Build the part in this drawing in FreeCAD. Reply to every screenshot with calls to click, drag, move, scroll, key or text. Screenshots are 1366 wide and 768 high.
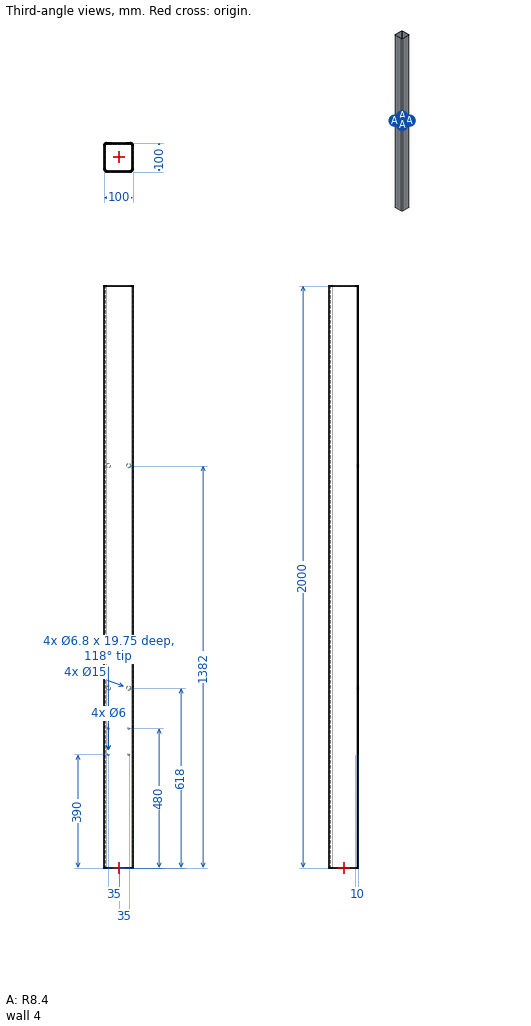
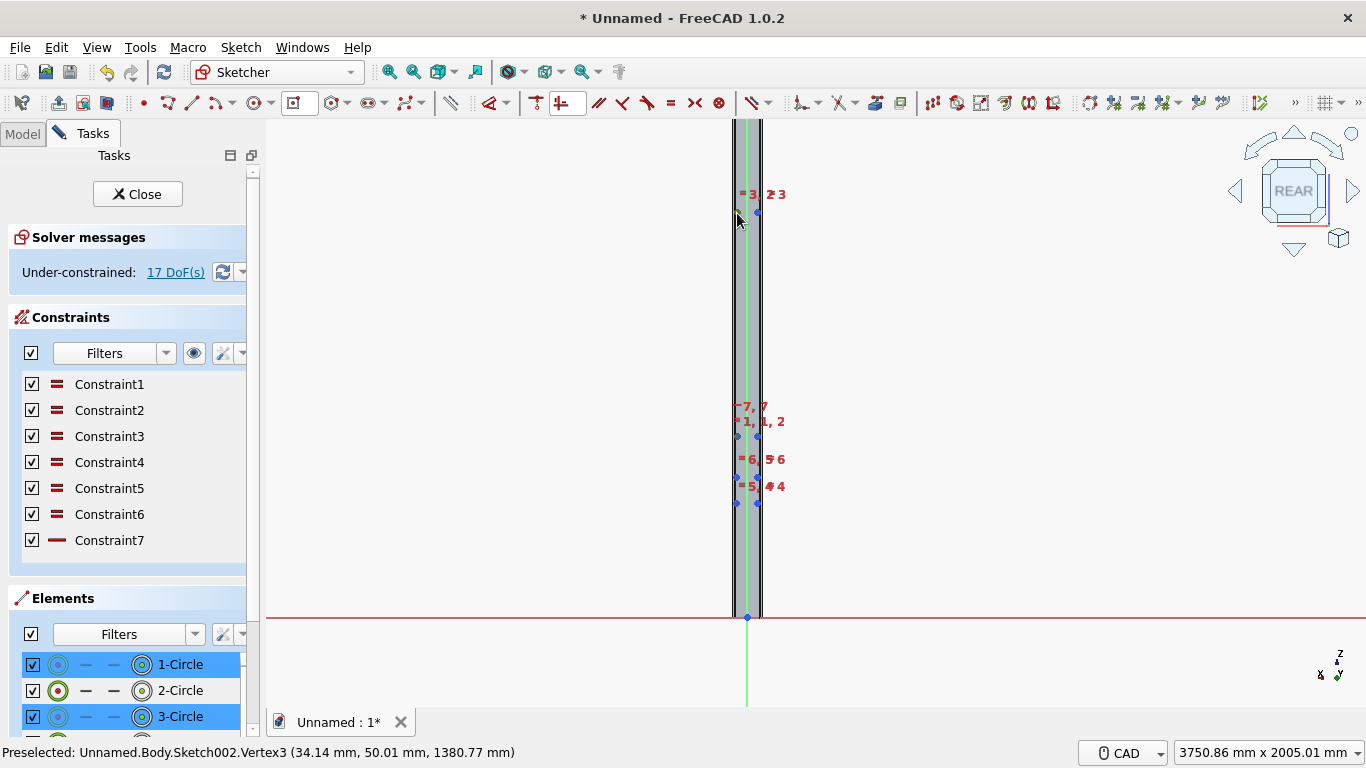
key(v)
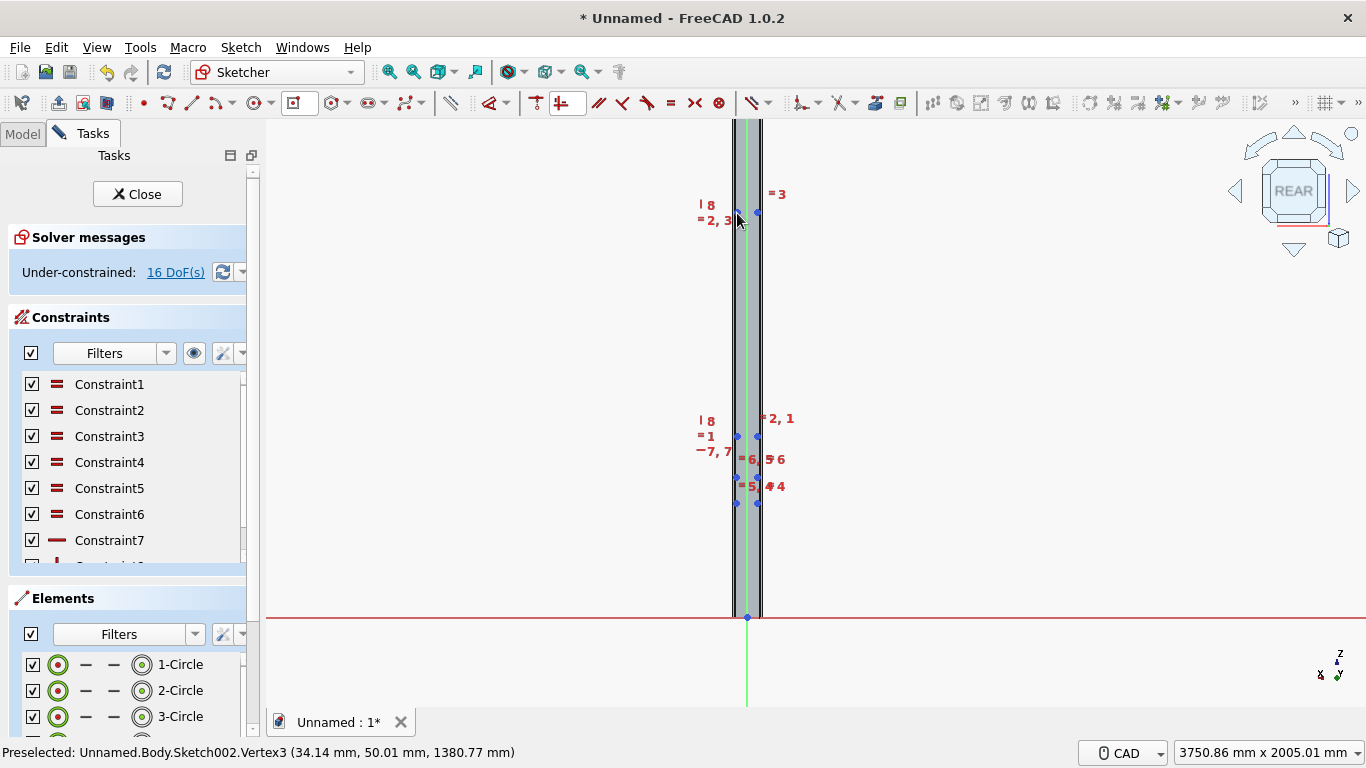
click(758, 437)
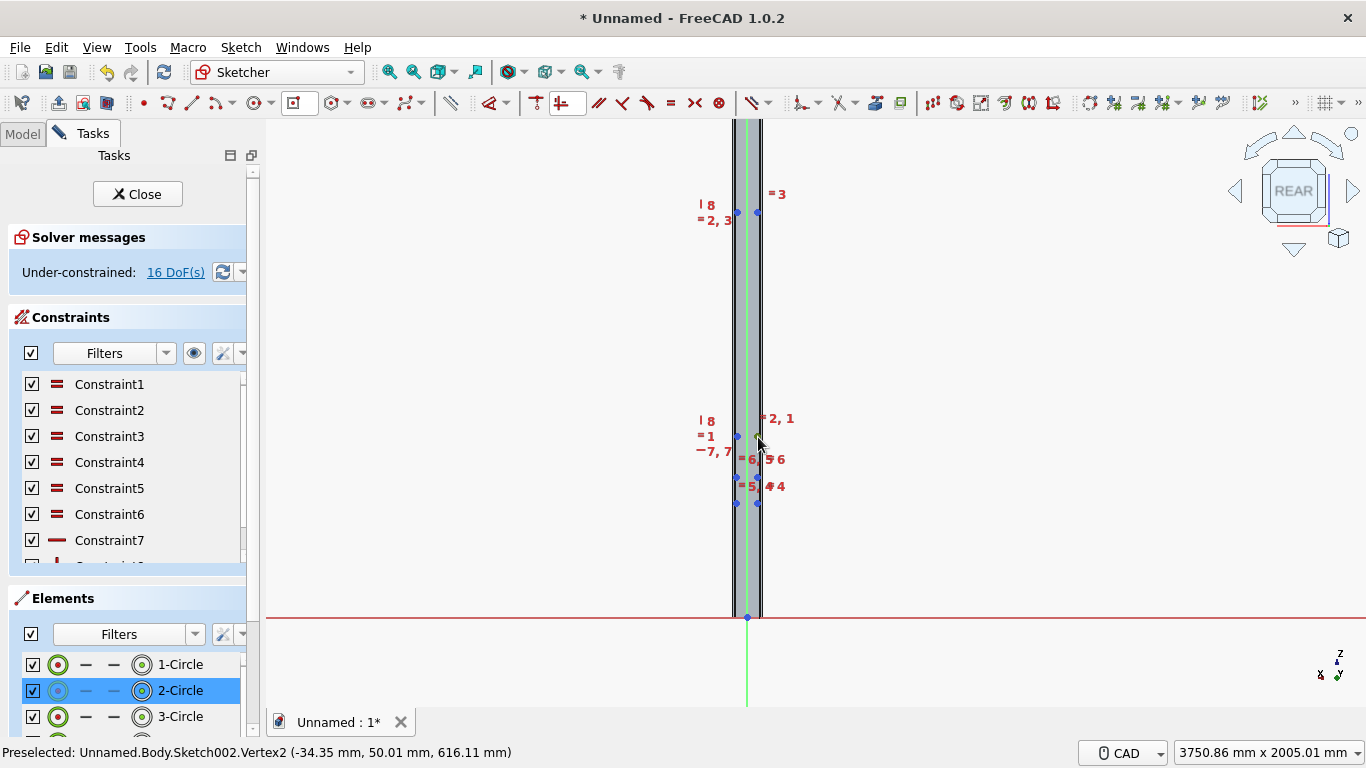
click(758, 213)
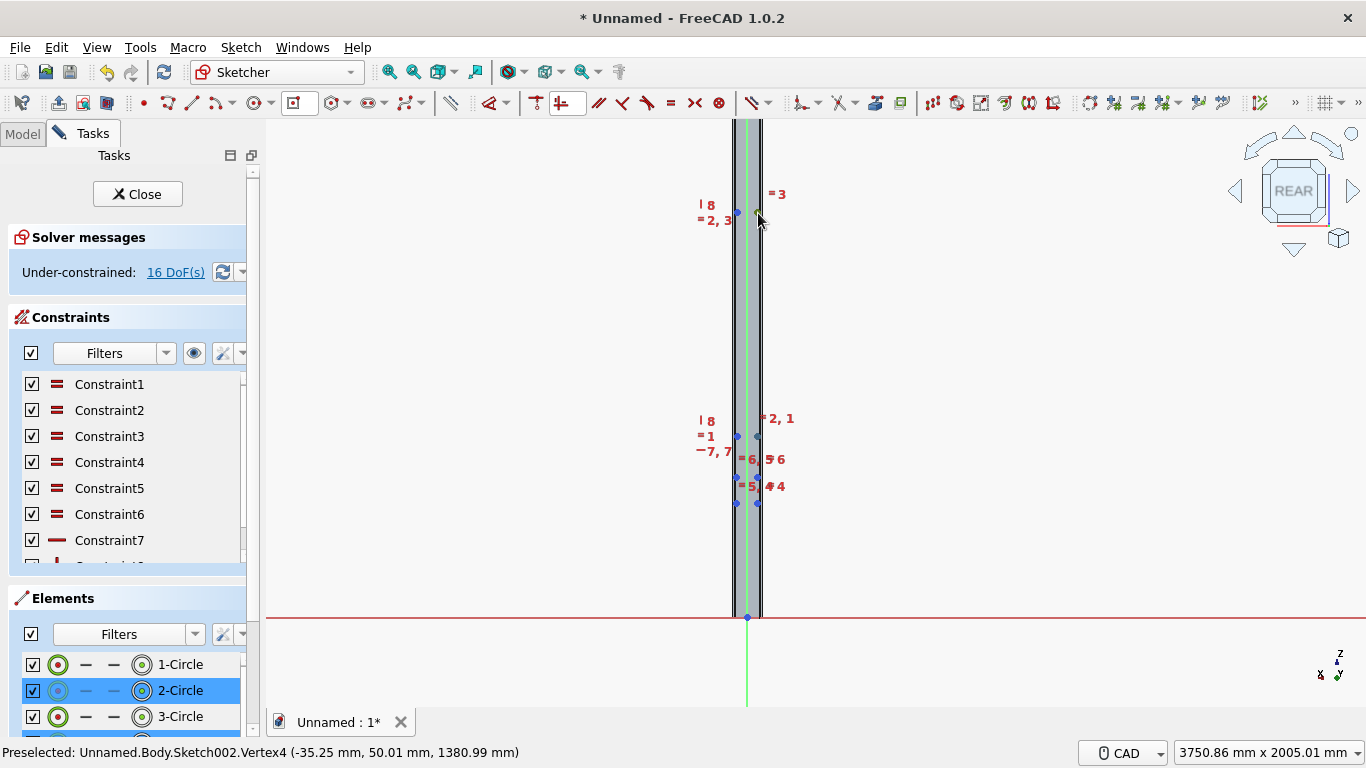
click(580, 104)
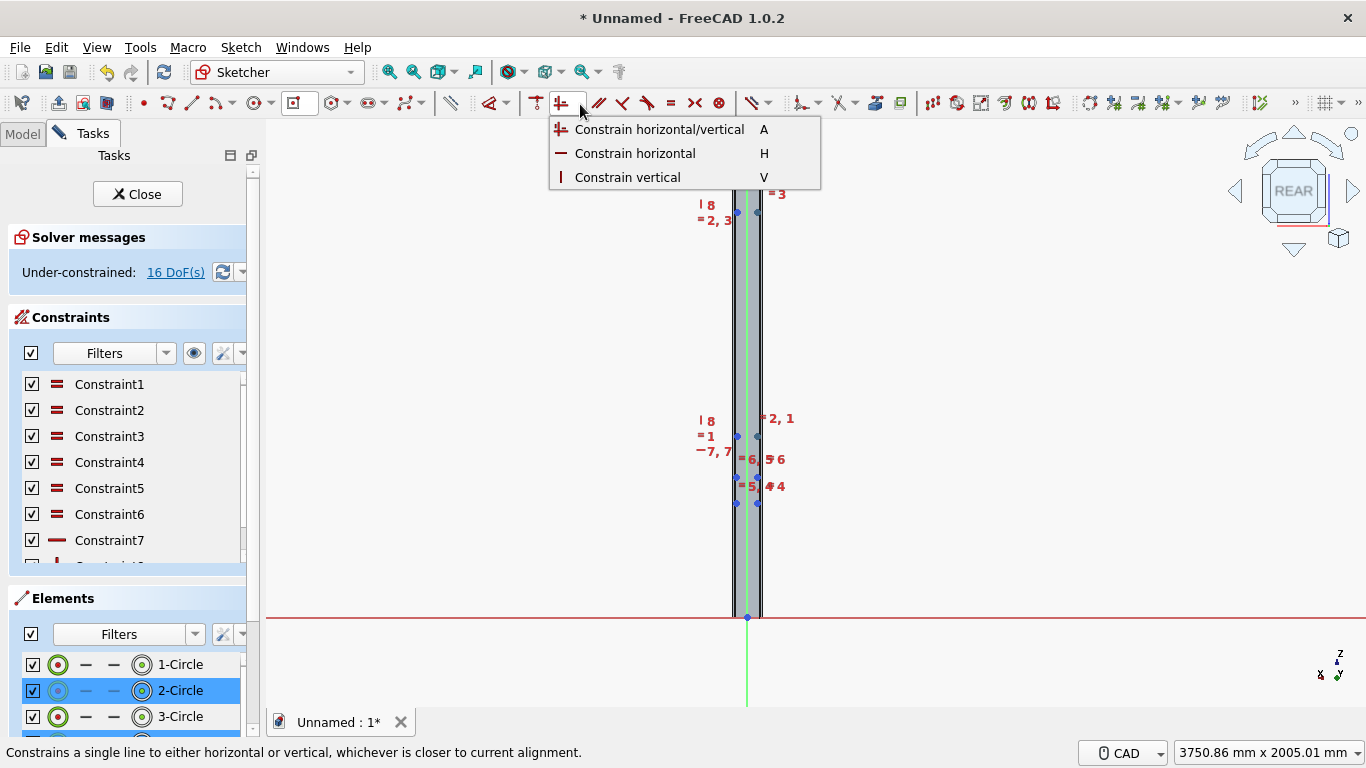
click(685, 177)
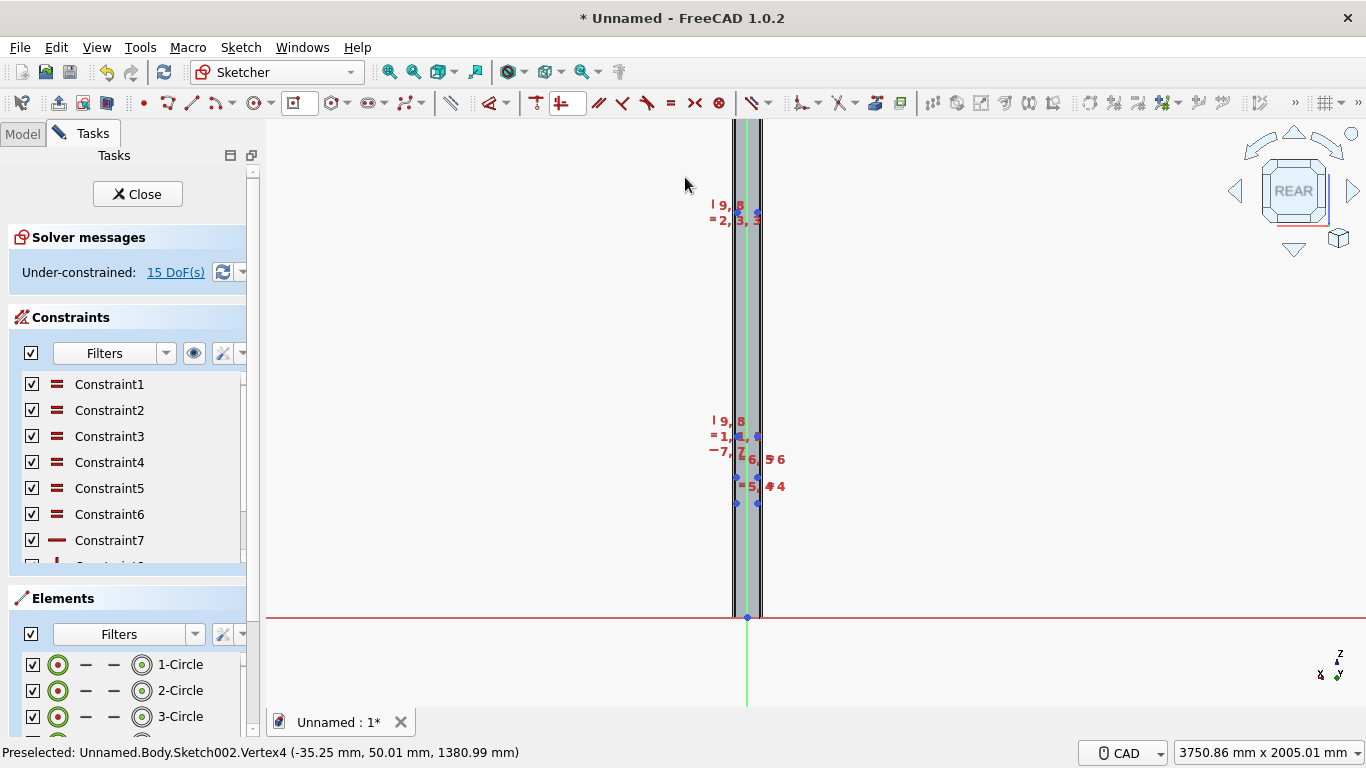
scroll(737, 213, up, 4)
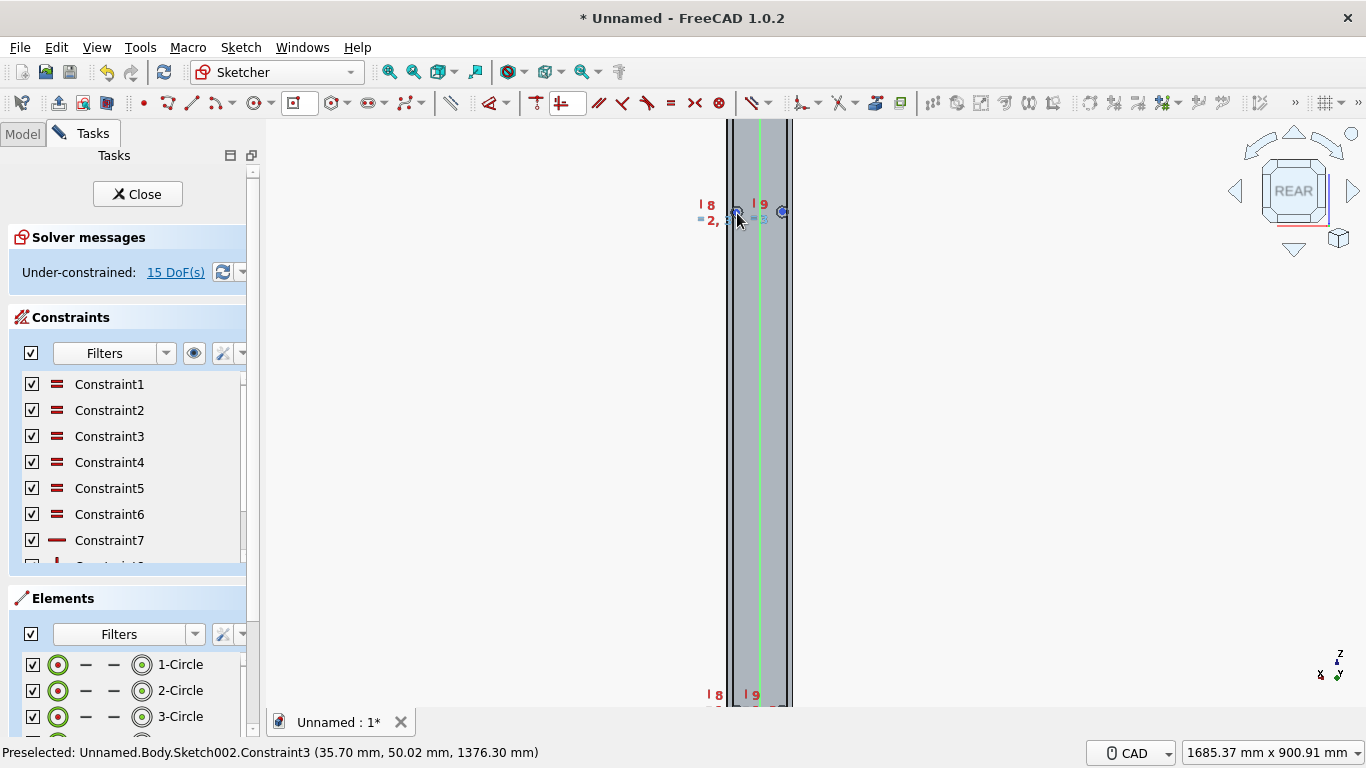
click(737, 212)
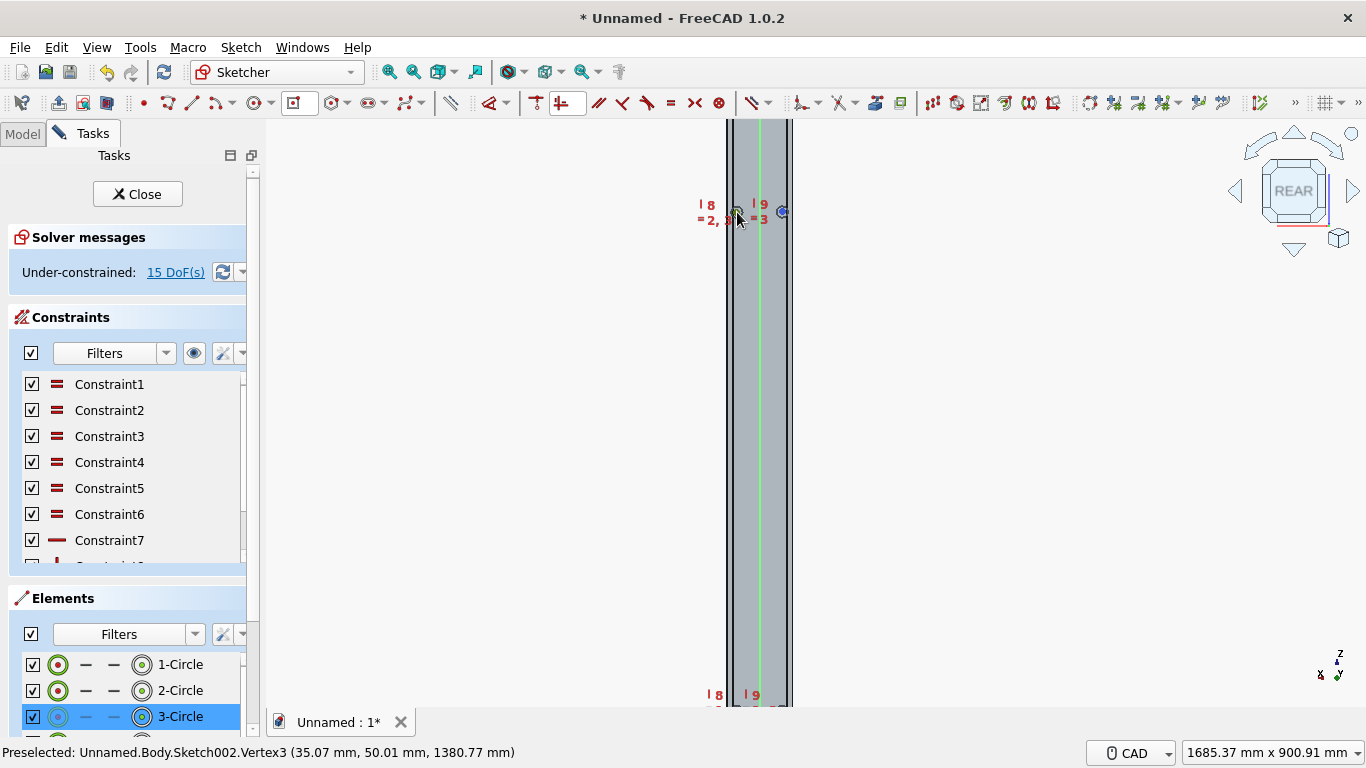
click(782, 212)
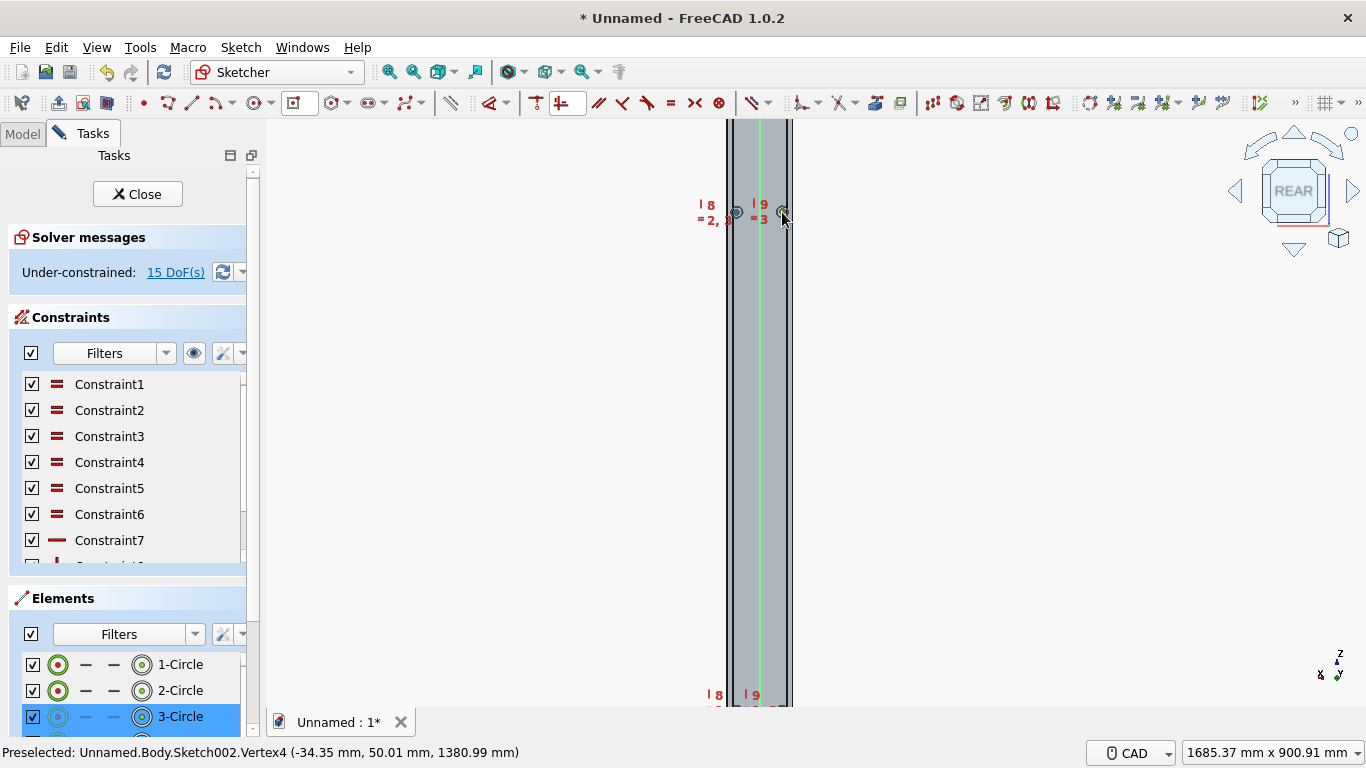
click(580, 104)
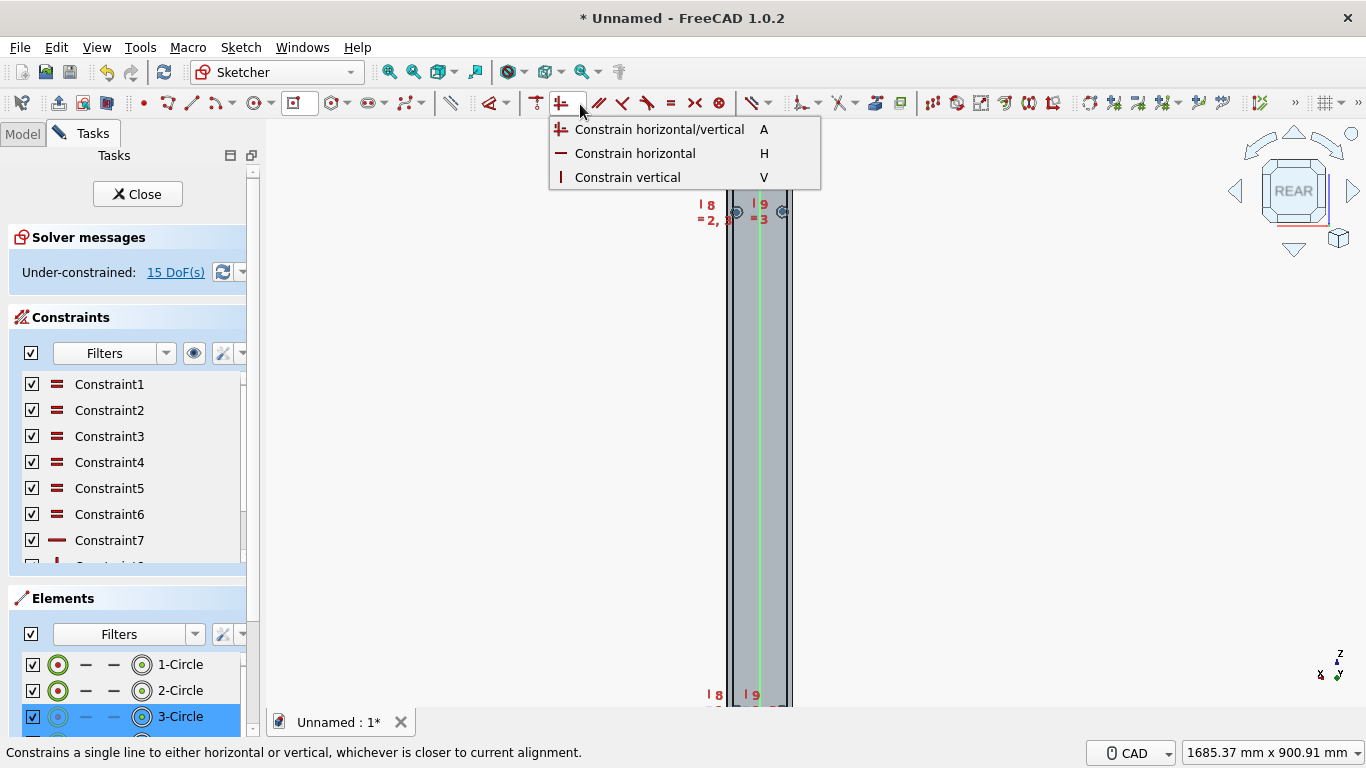
click(685, 153)